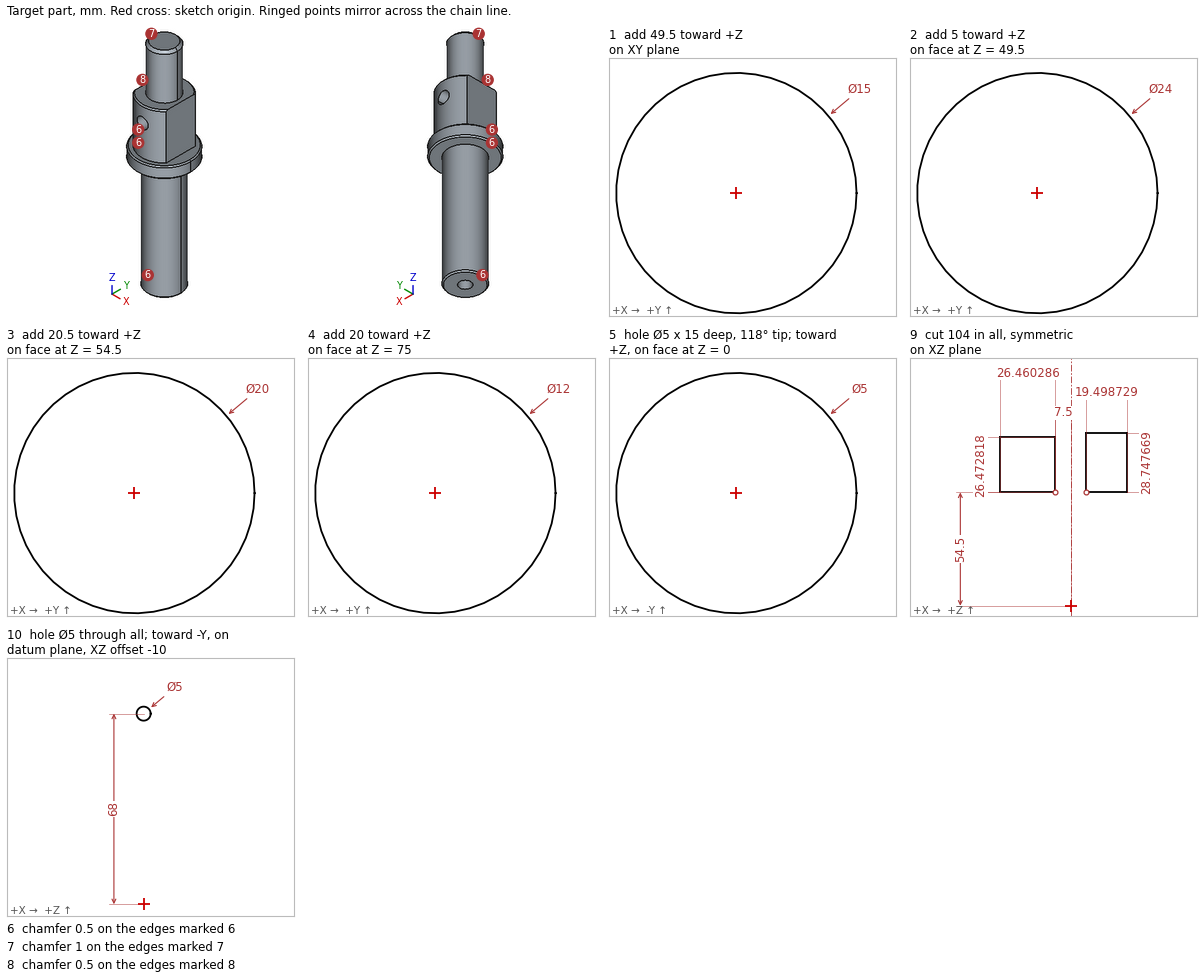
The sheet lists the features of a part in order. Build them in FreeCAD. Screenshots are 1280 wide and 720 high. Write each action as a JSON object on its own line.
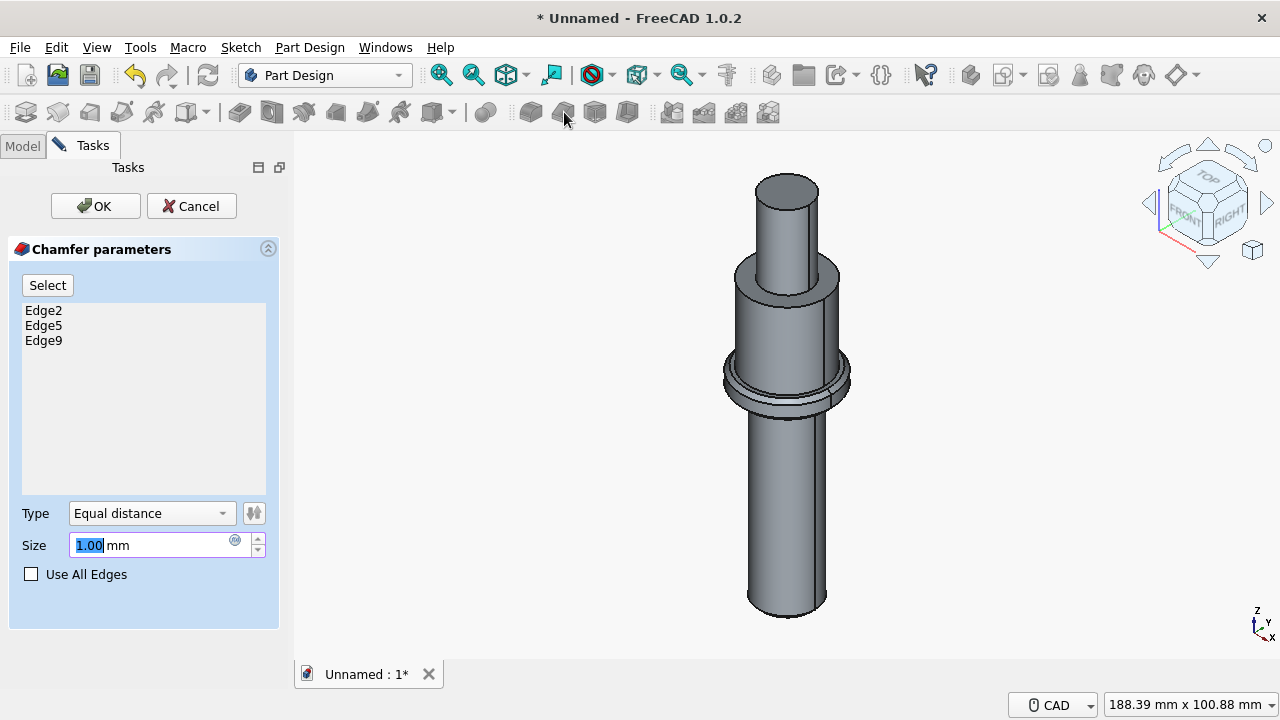
{"action": "type", "text": "0.5"}
{"action": "key", "text": "Tab"}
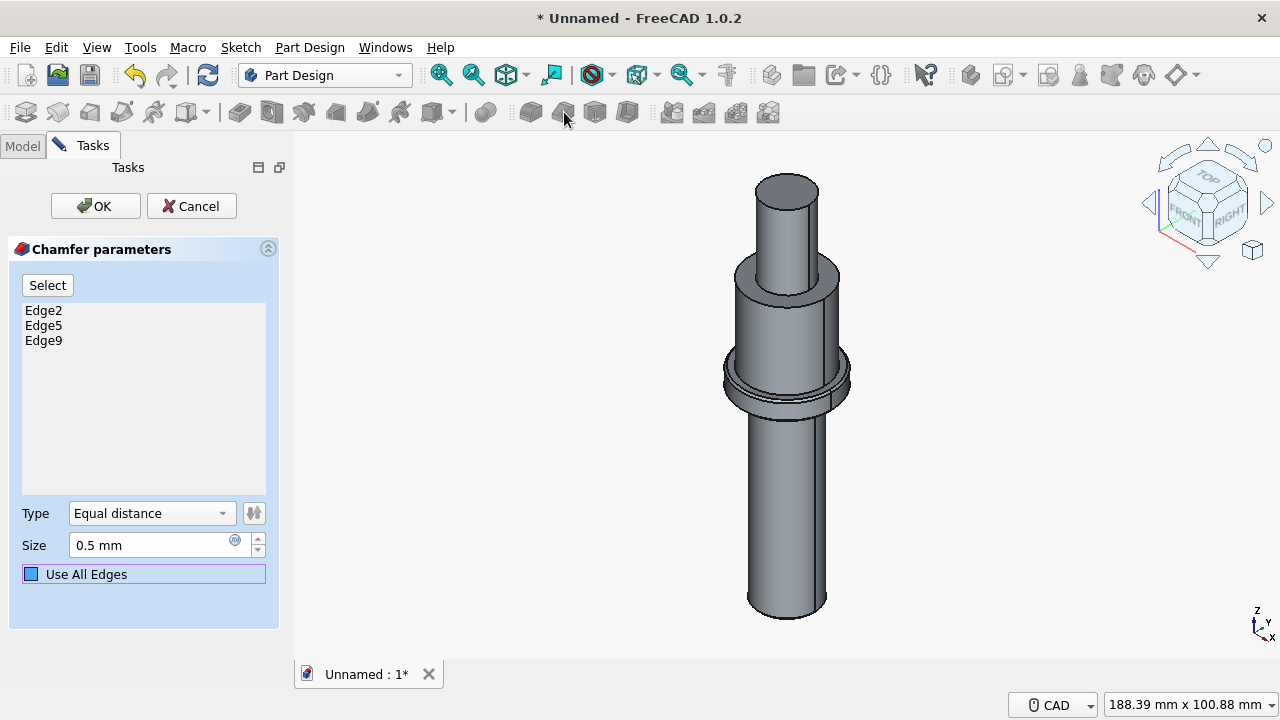
{"action": "left_click", "coordinate": [96, 206]}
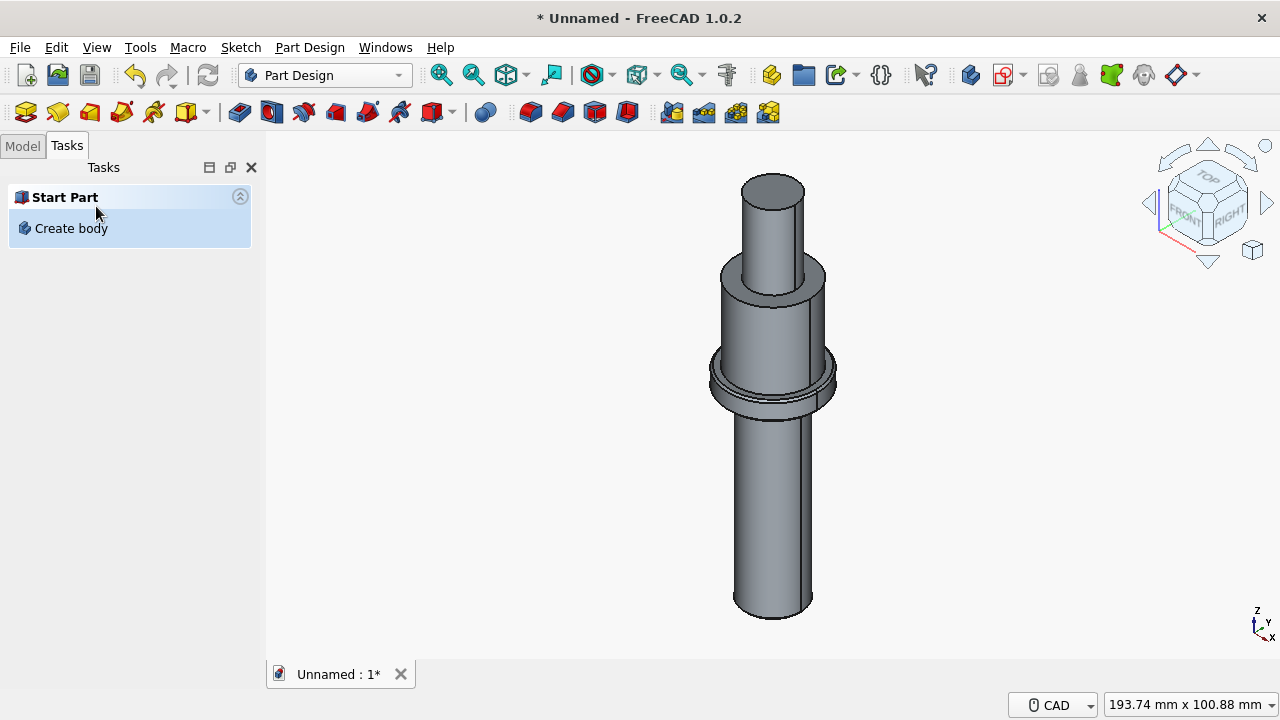
{"action": "left_click", "coordinate": [745, 199]}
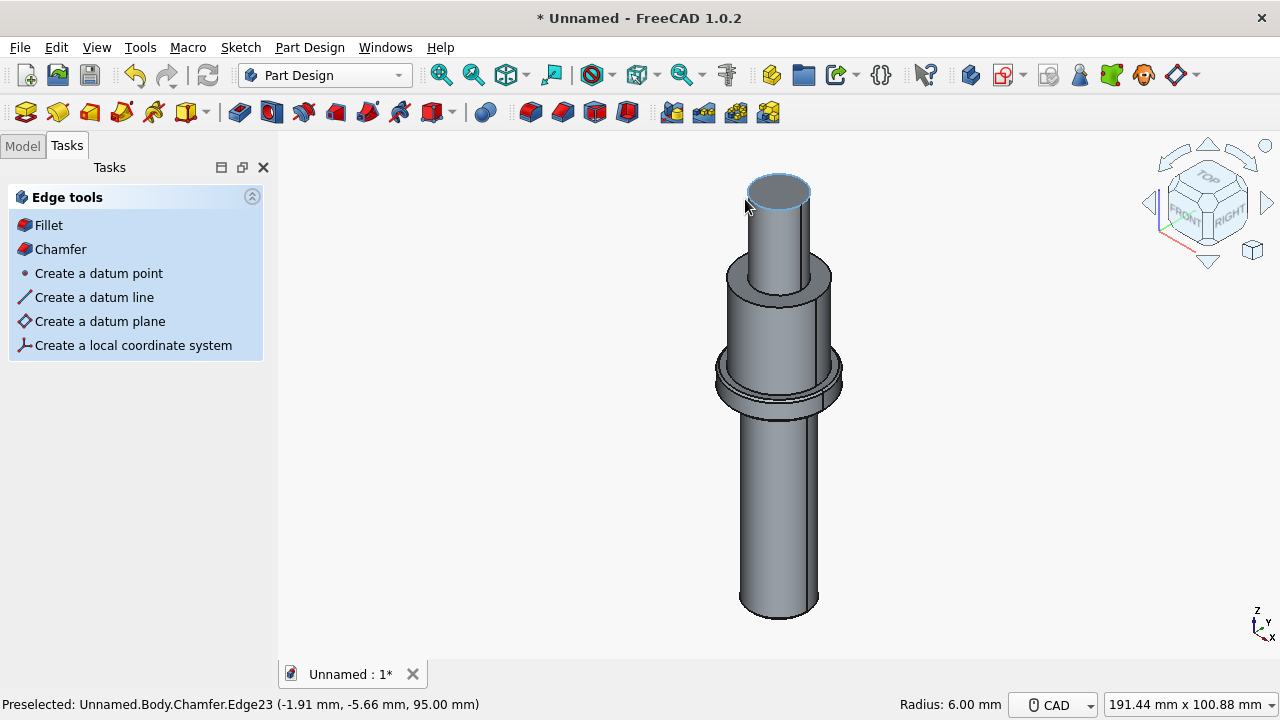
{"action": "left_click", "coordinate": [564, 112]}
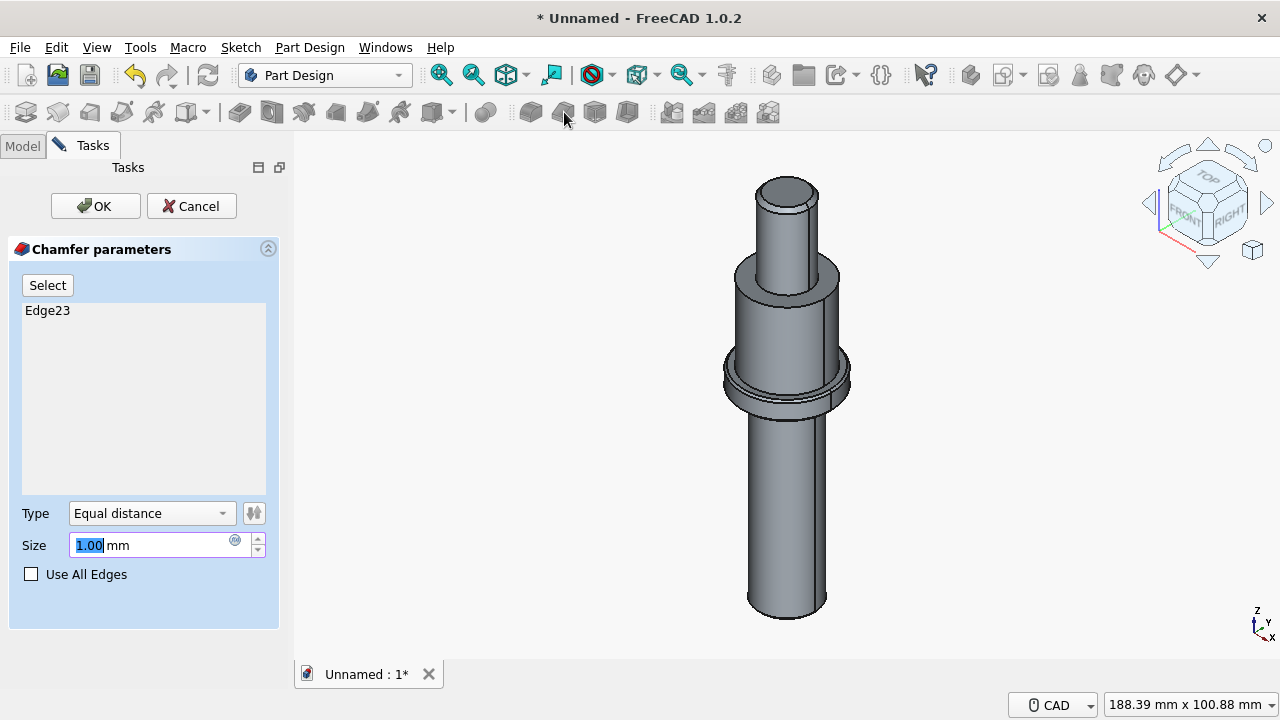
{"action": "type", "text": "1"}
{"action": "key", "text": "Tab"}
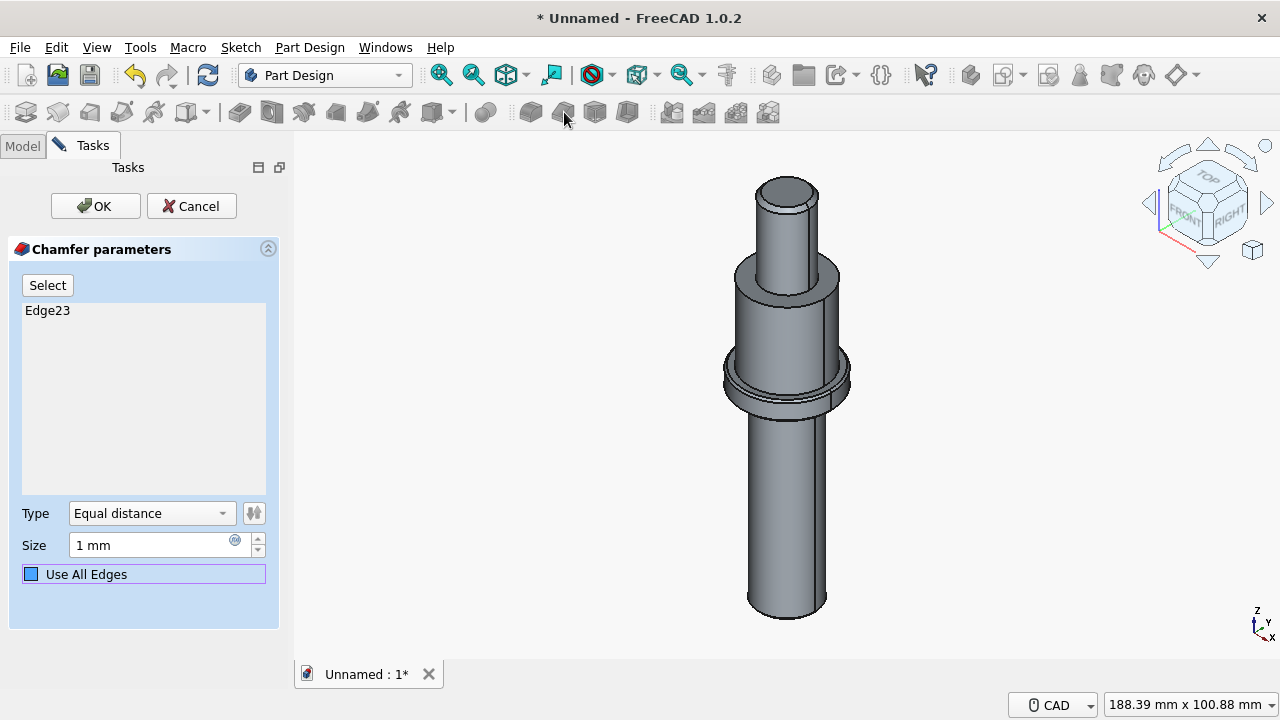
{"action": "left_click", "coordinate": [96, 206]}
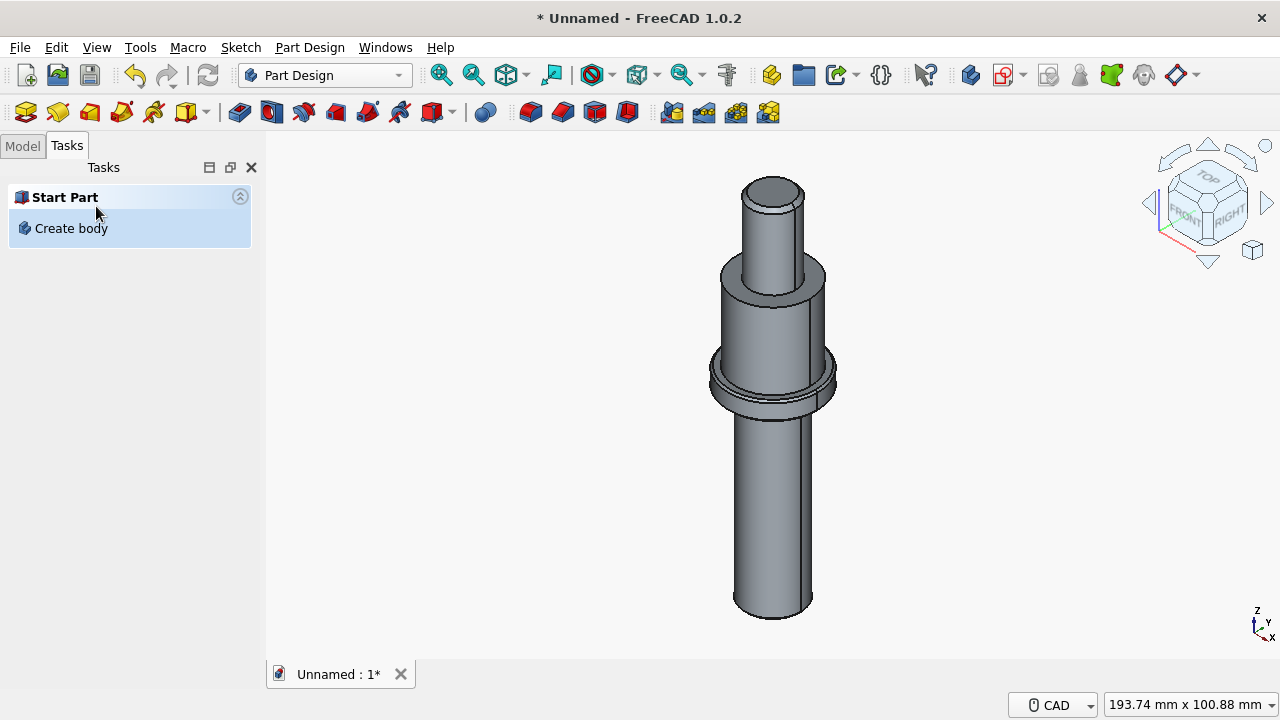
{"action": "left_click", "coordinate": [726, 290]}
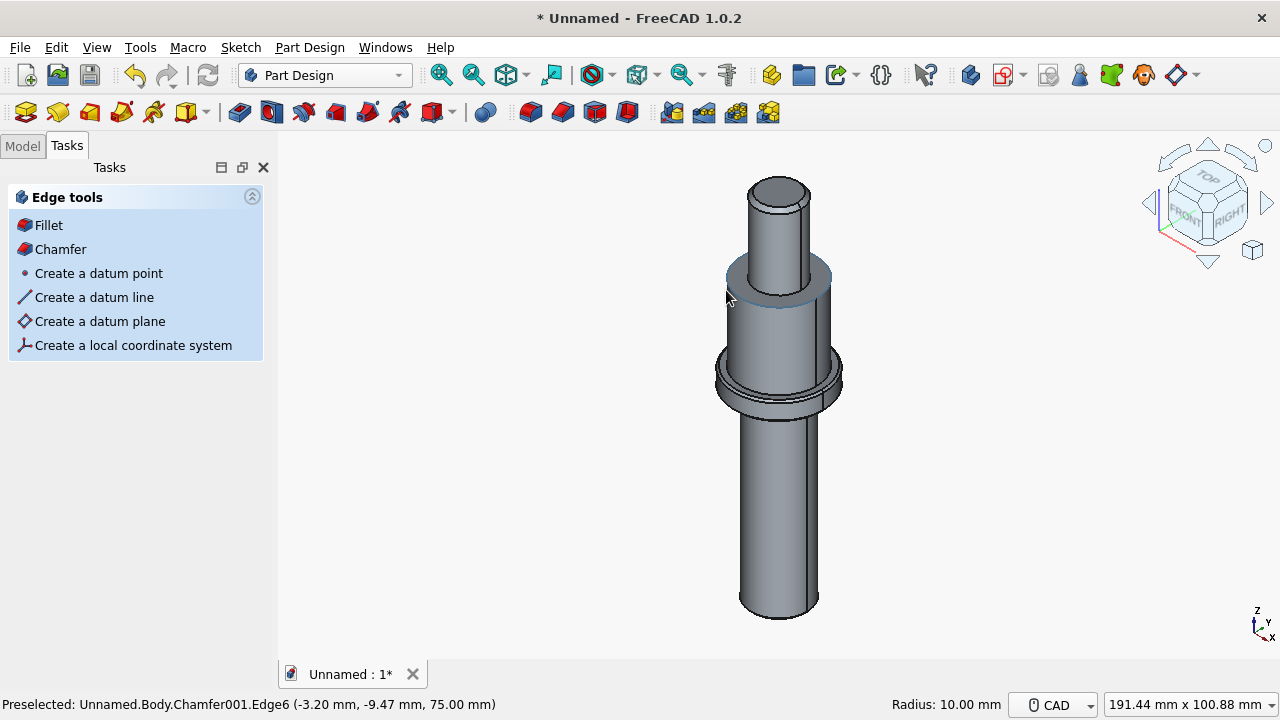
{"action": "left_click", "coordinate": [564, 112]}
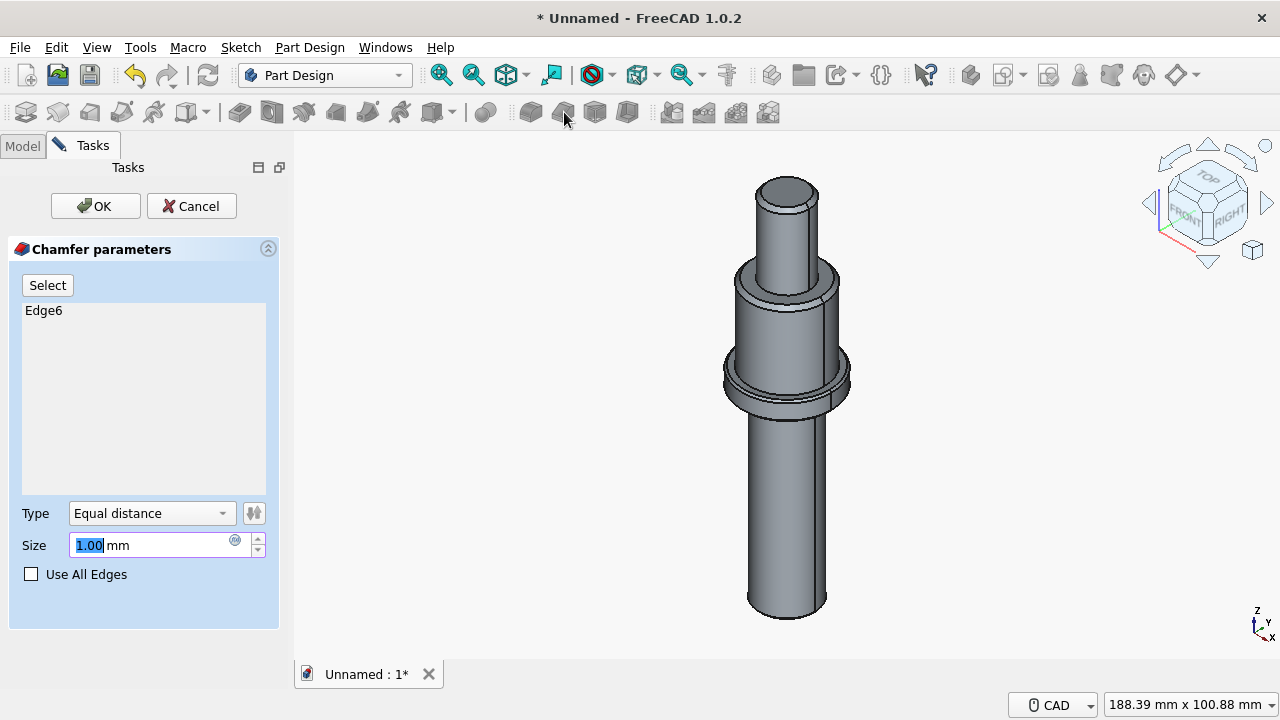
{"action": "type", "text": "0.5"}
{"action": "key", "text": "Tab"}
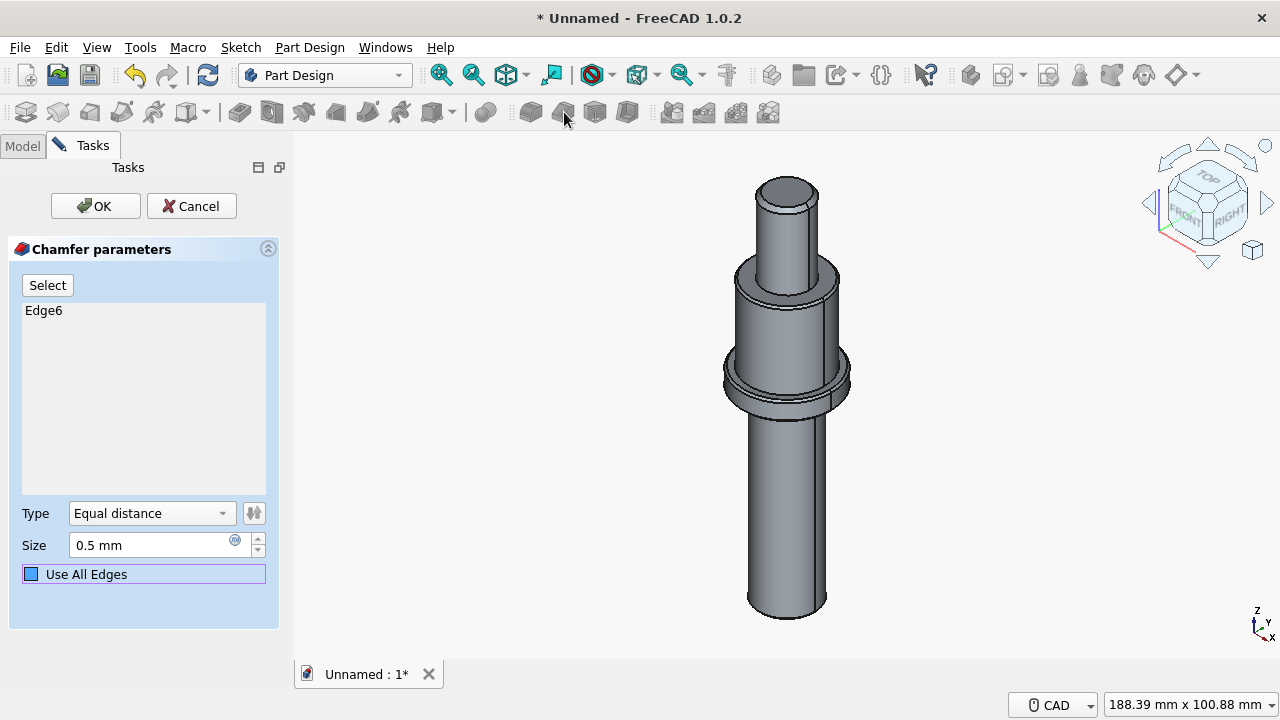
{"action": "left_click", "coordinate": [96, 206]}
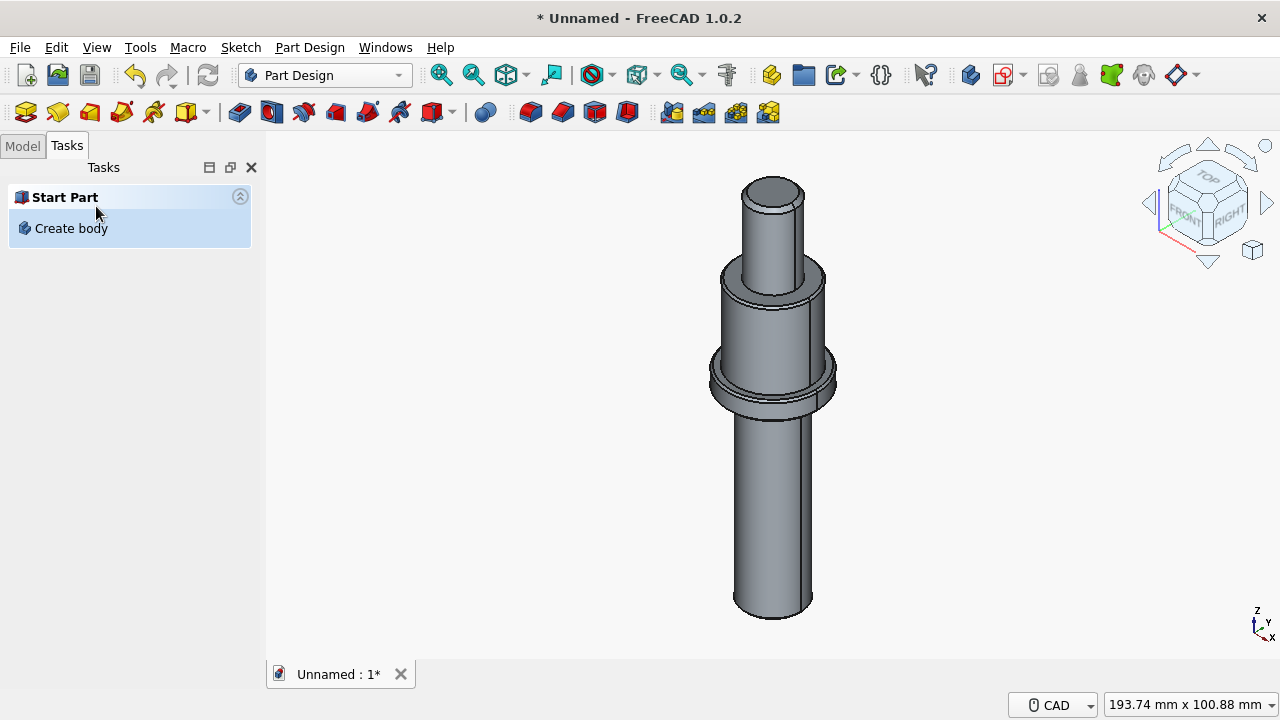
{"action": "left_click", "coordinate": [1004, 76]}